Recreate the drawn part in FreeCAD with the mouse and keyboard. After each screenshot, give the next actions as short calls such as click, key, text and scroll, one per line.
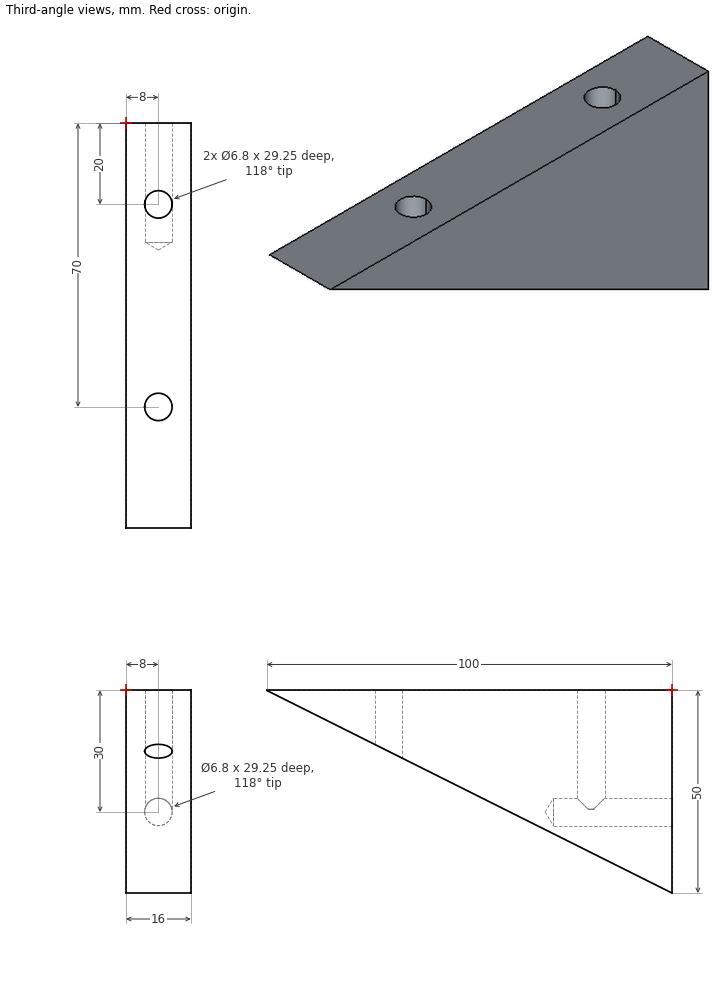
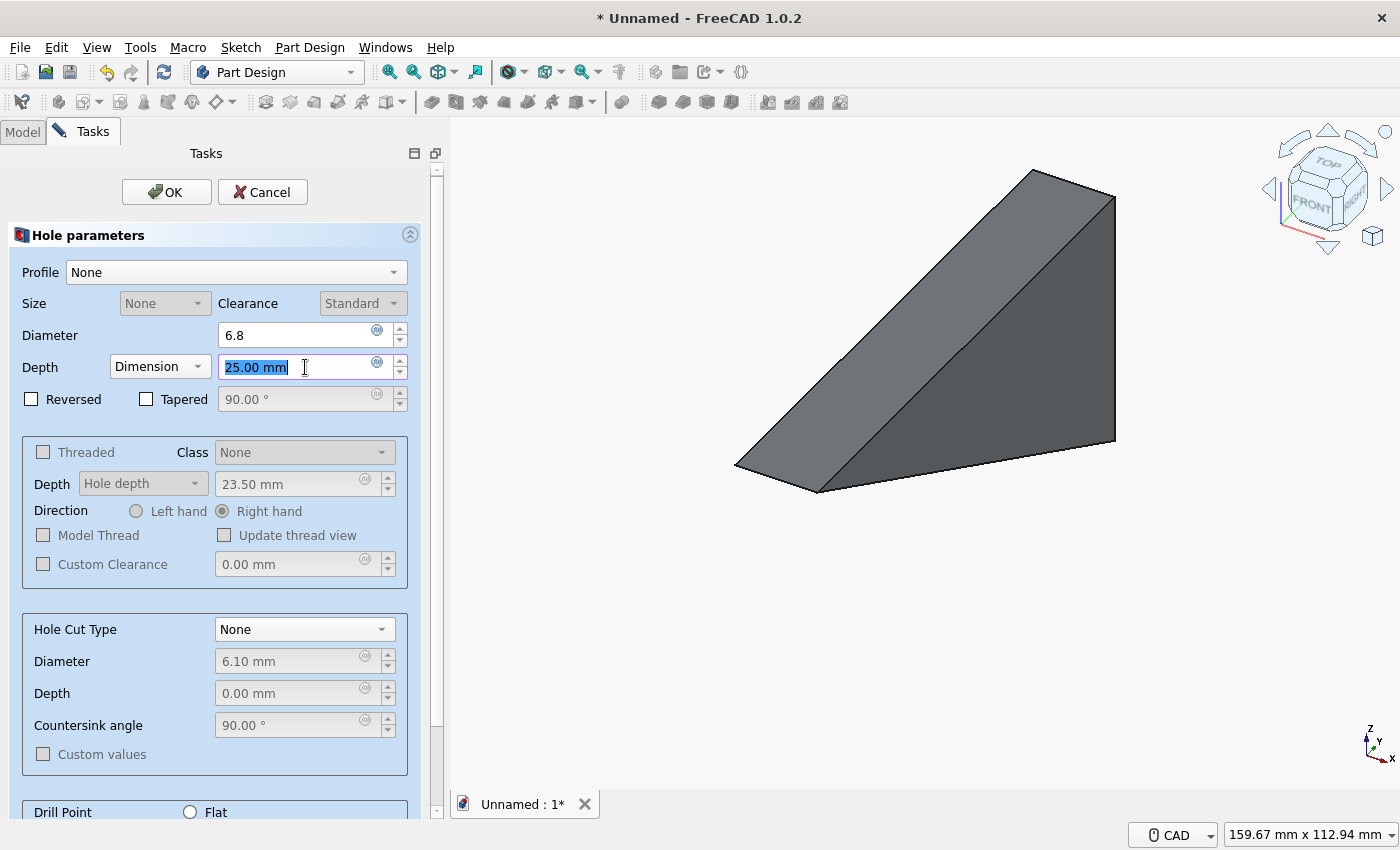
text(29.25)
key(Tab)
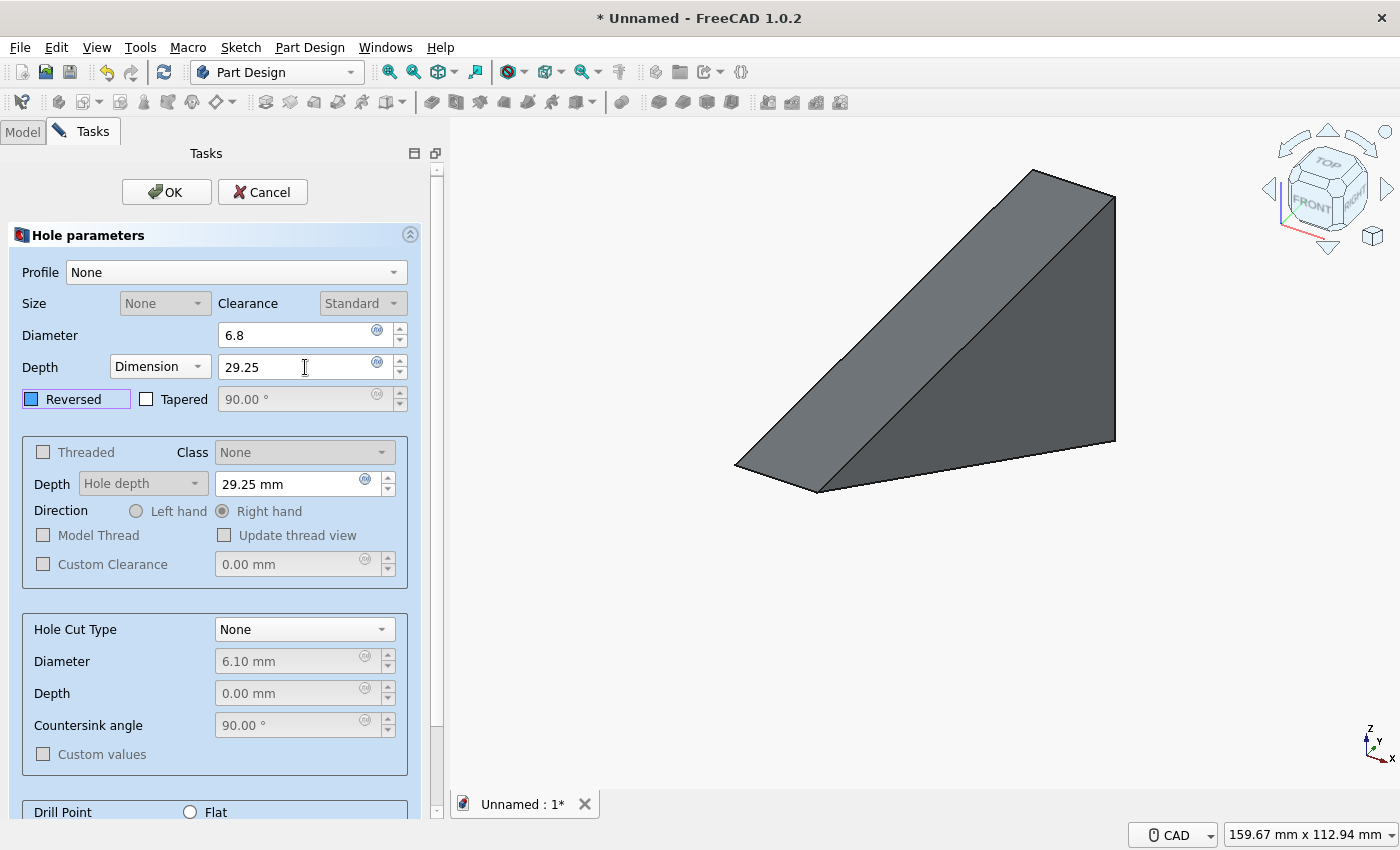
click(30, 399)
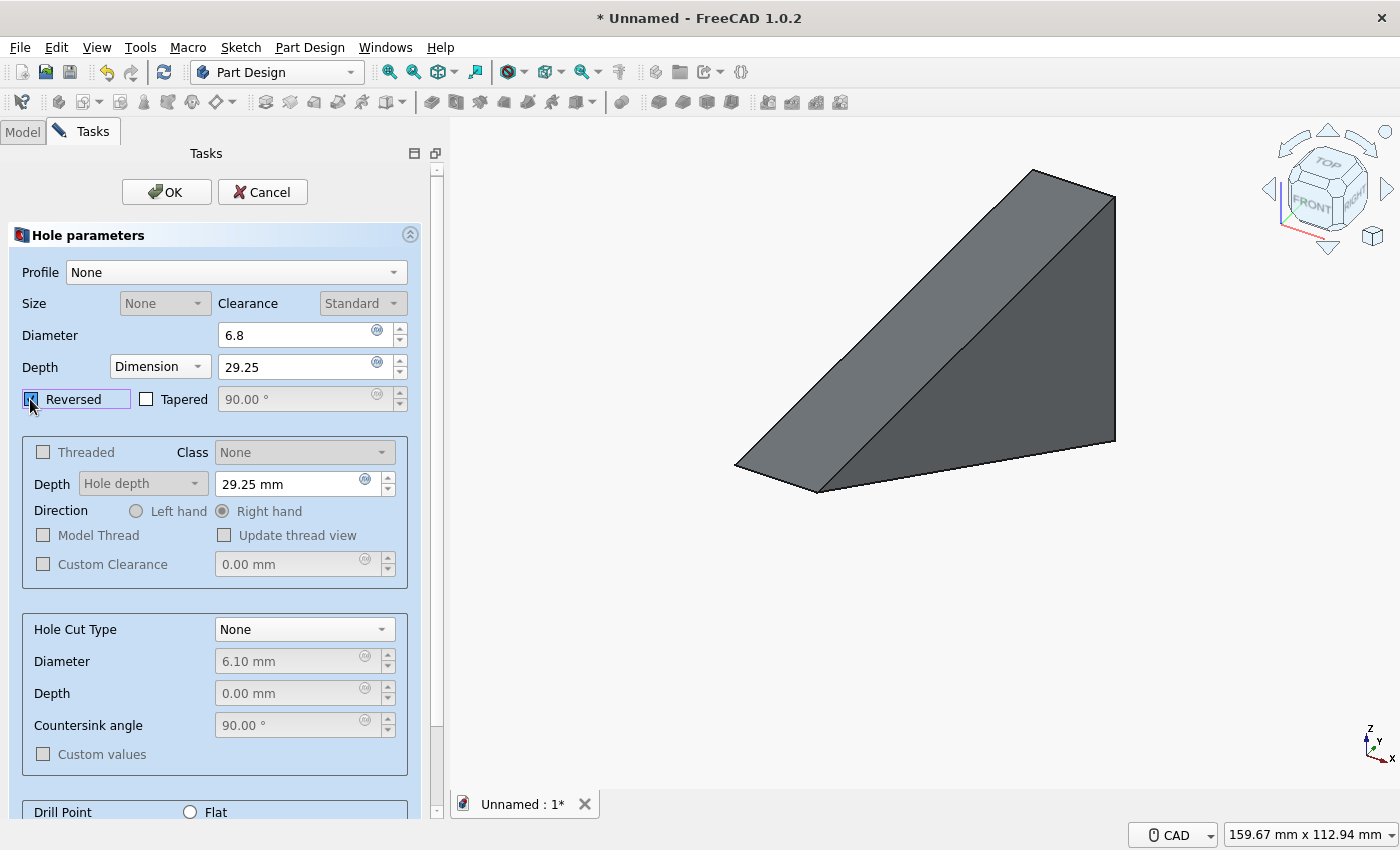
click(167, 192)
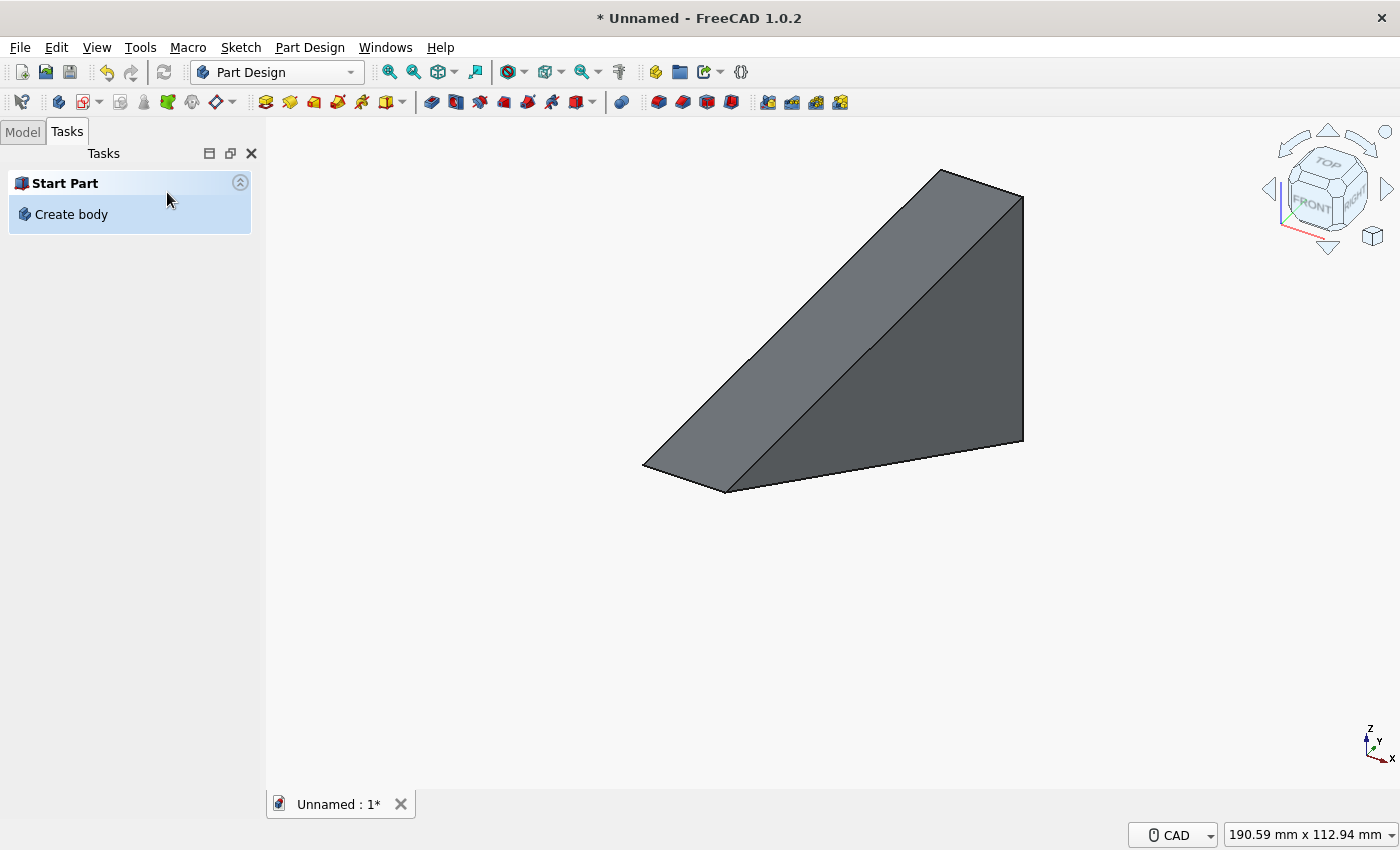
click(84, 102)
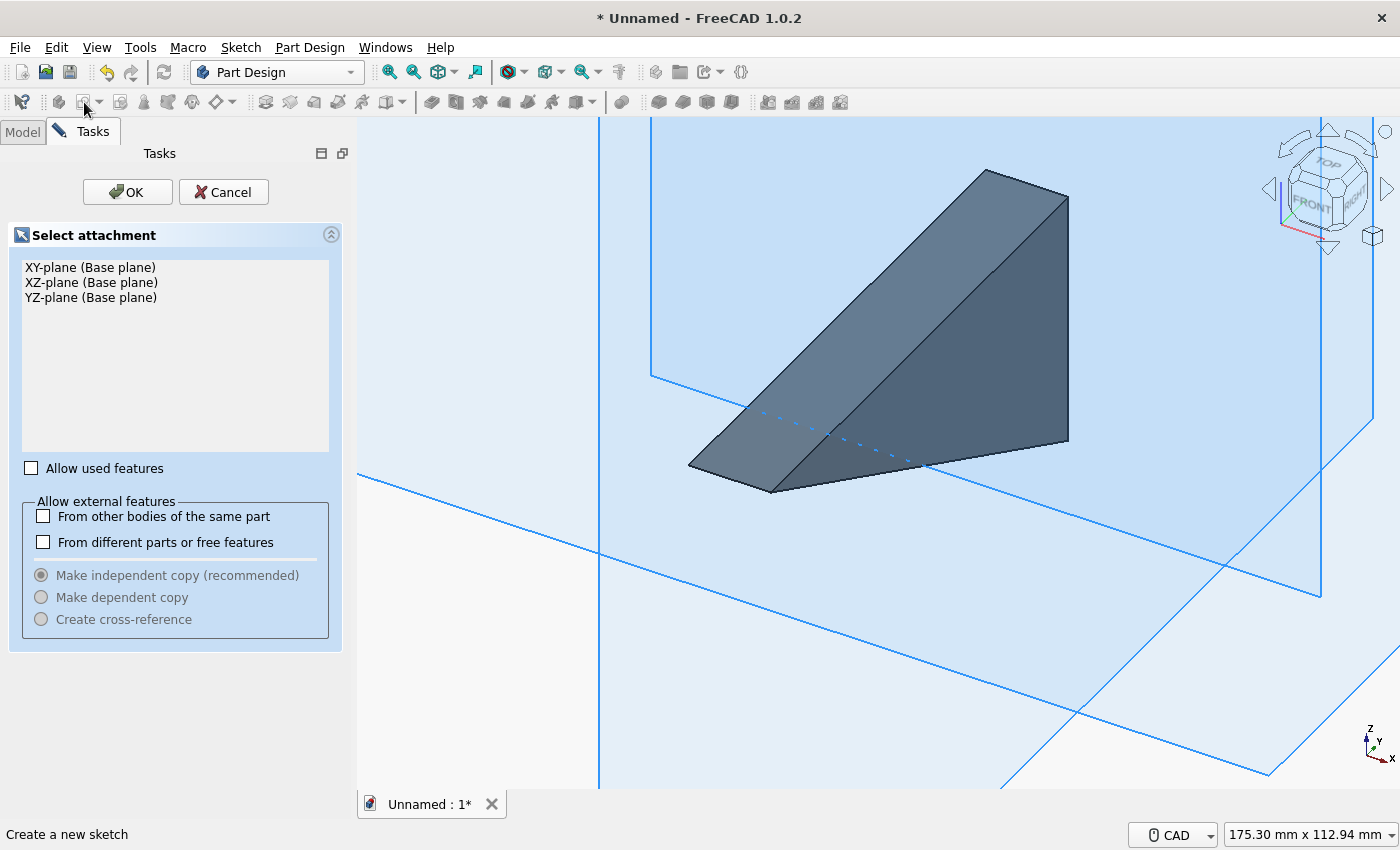
click(82, 268)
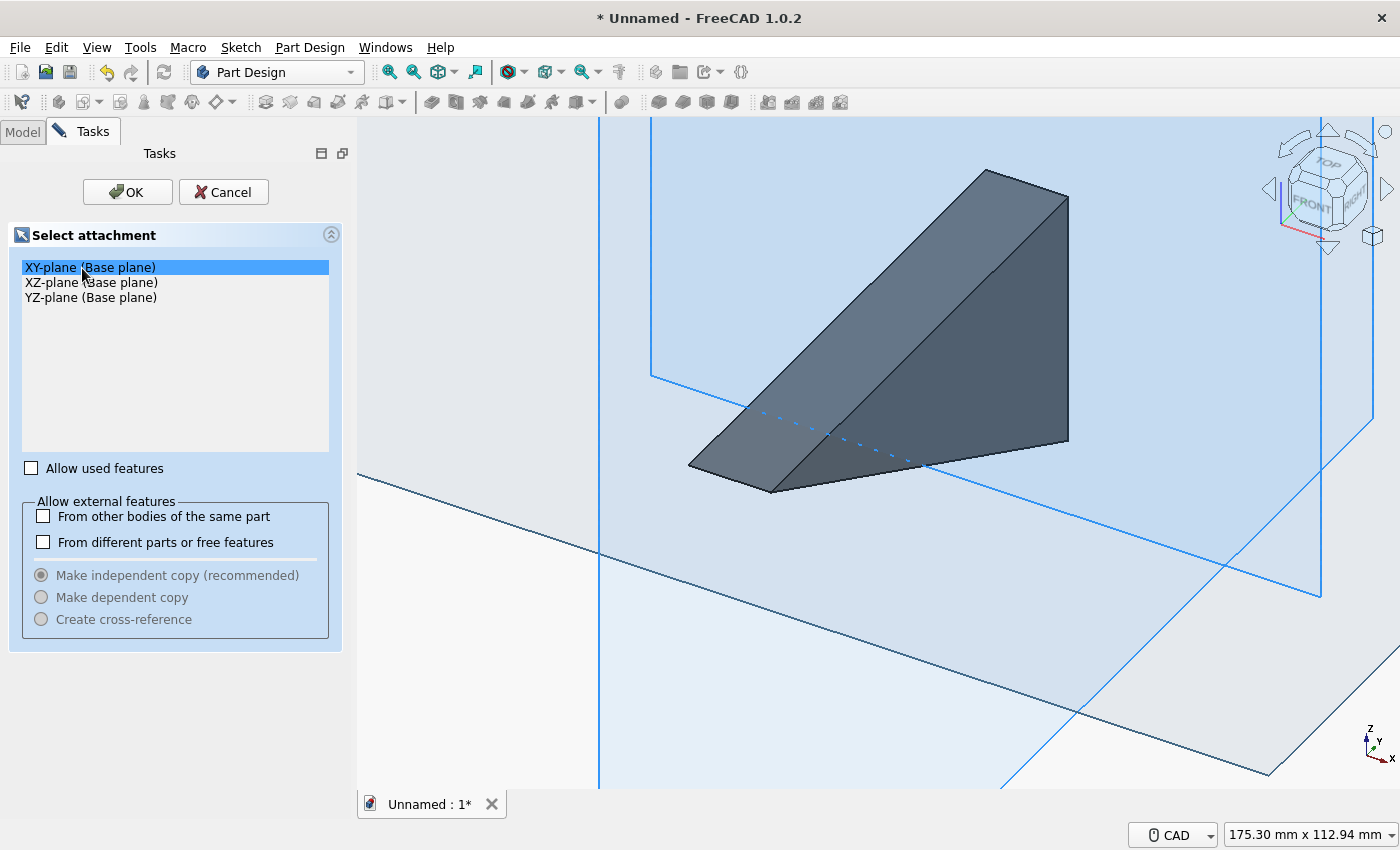
click(128, 192)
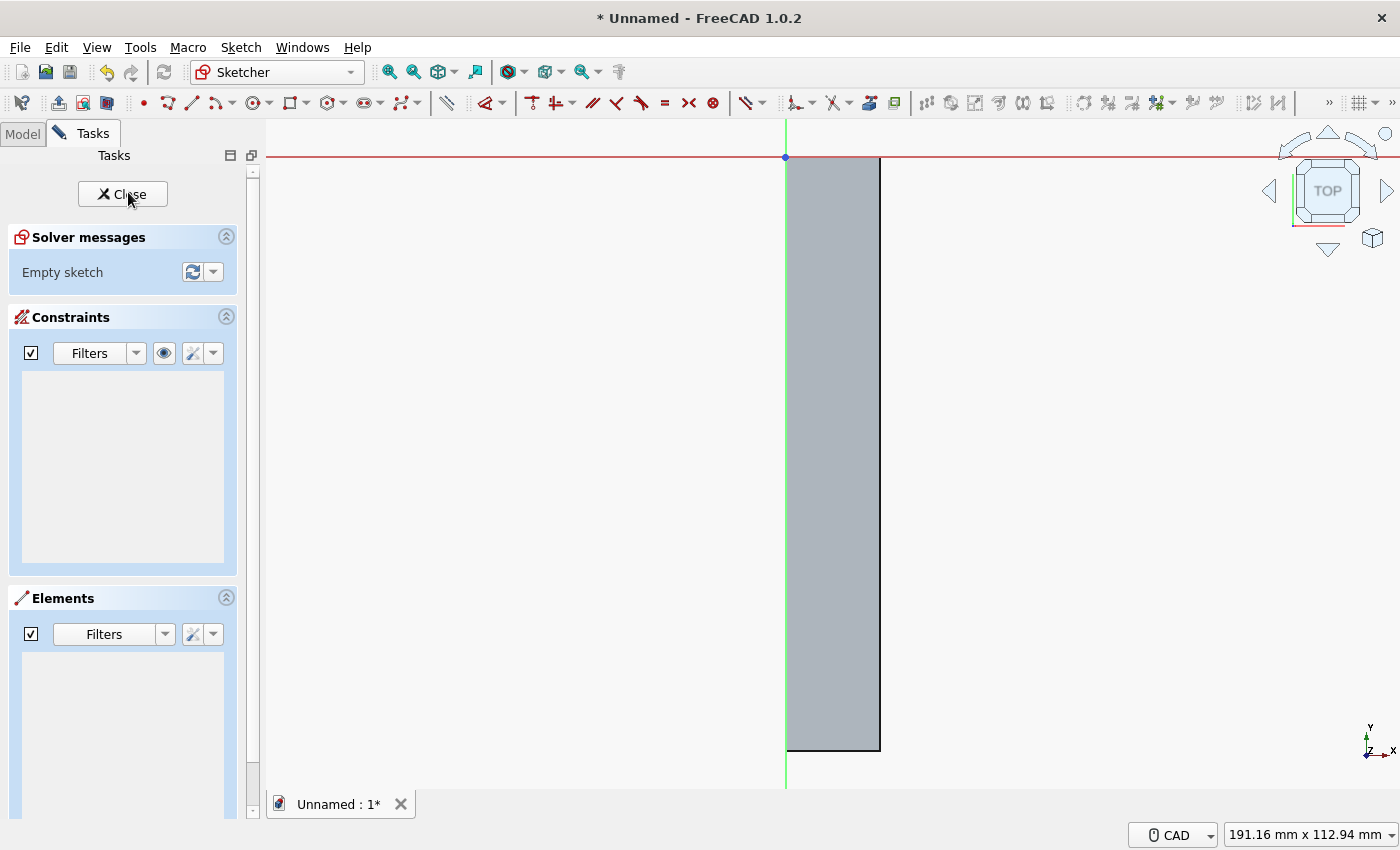
scroll(517, 761, down, 1)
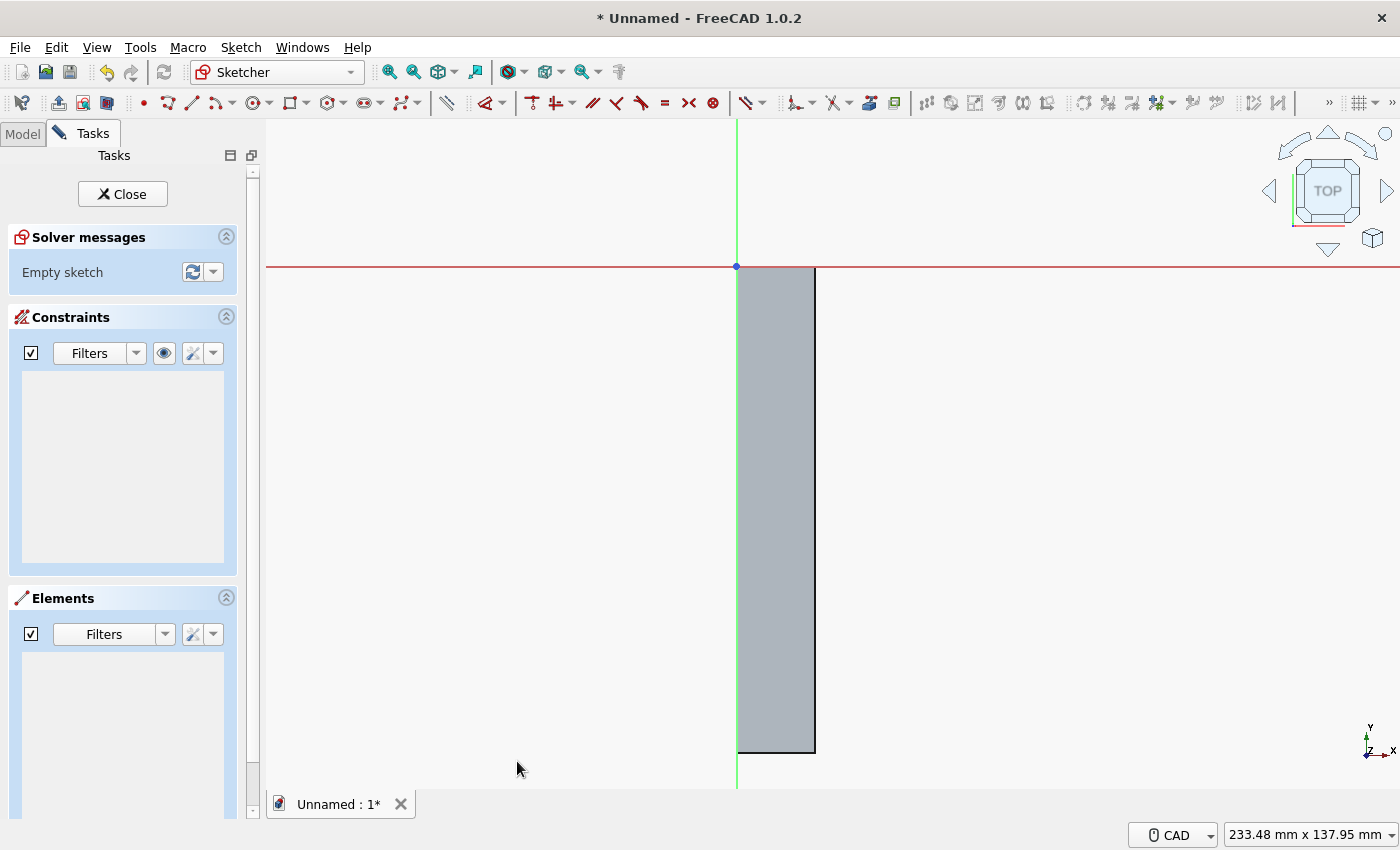
click(254, 104)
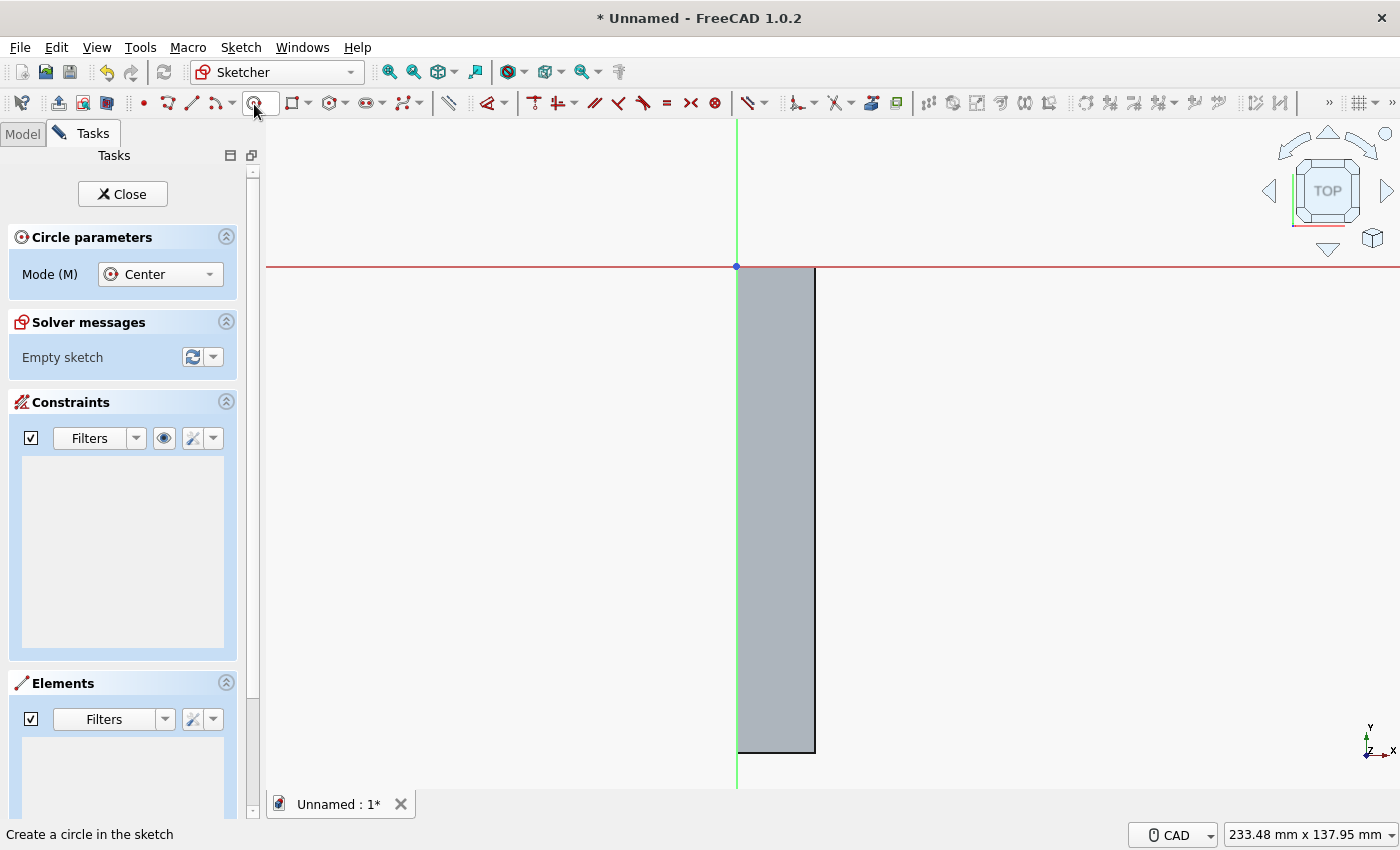
scroll(776, 364, up, 2)